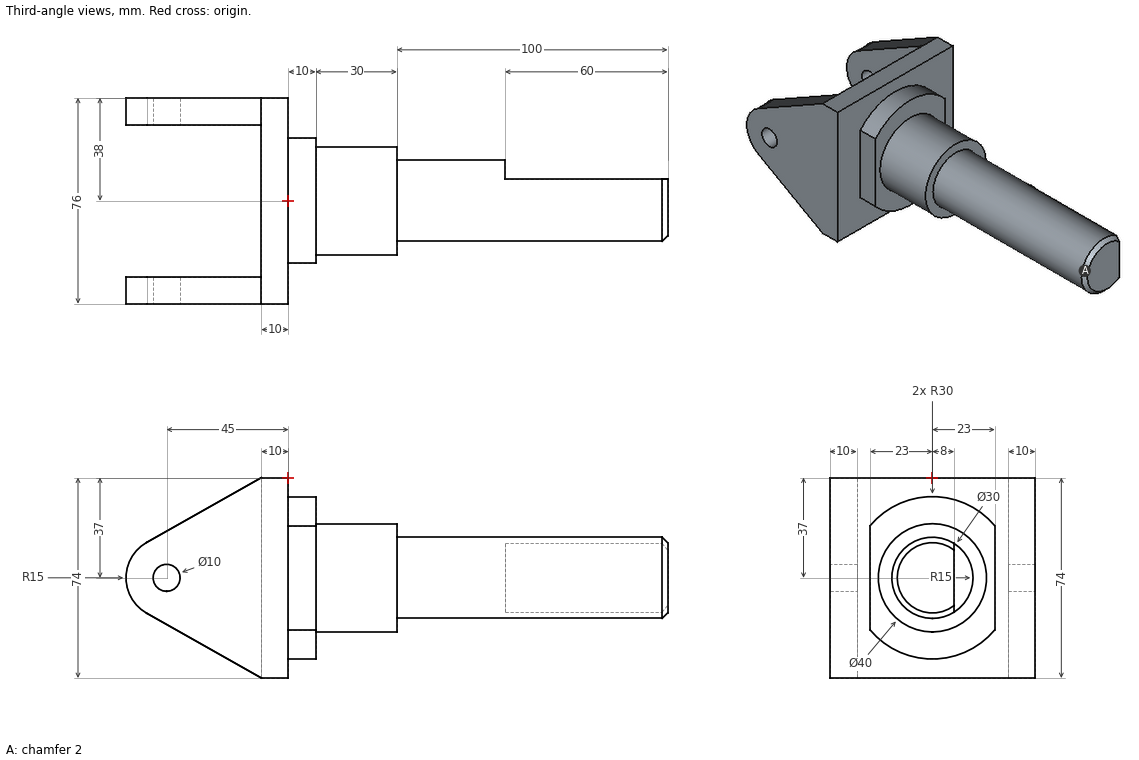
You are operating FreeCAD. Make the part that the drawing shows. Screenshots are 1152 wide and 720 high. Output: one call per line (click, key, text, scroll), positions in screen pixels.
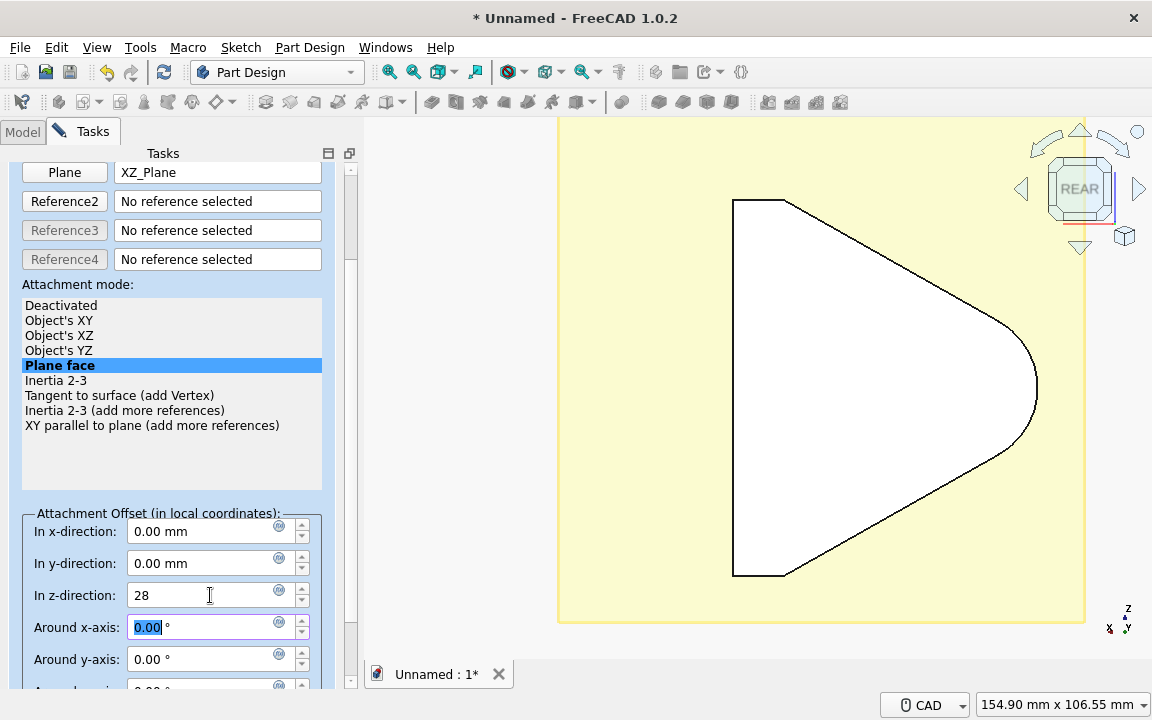
scroll(351, 426, up, 3)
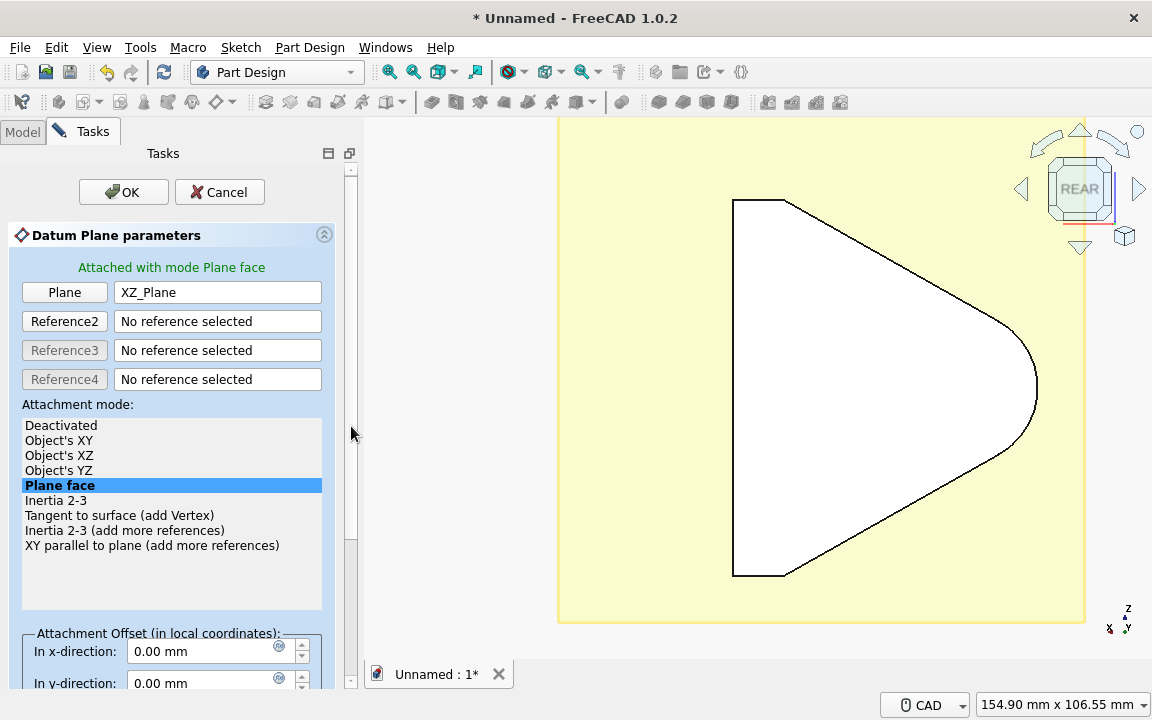
click(124, 192)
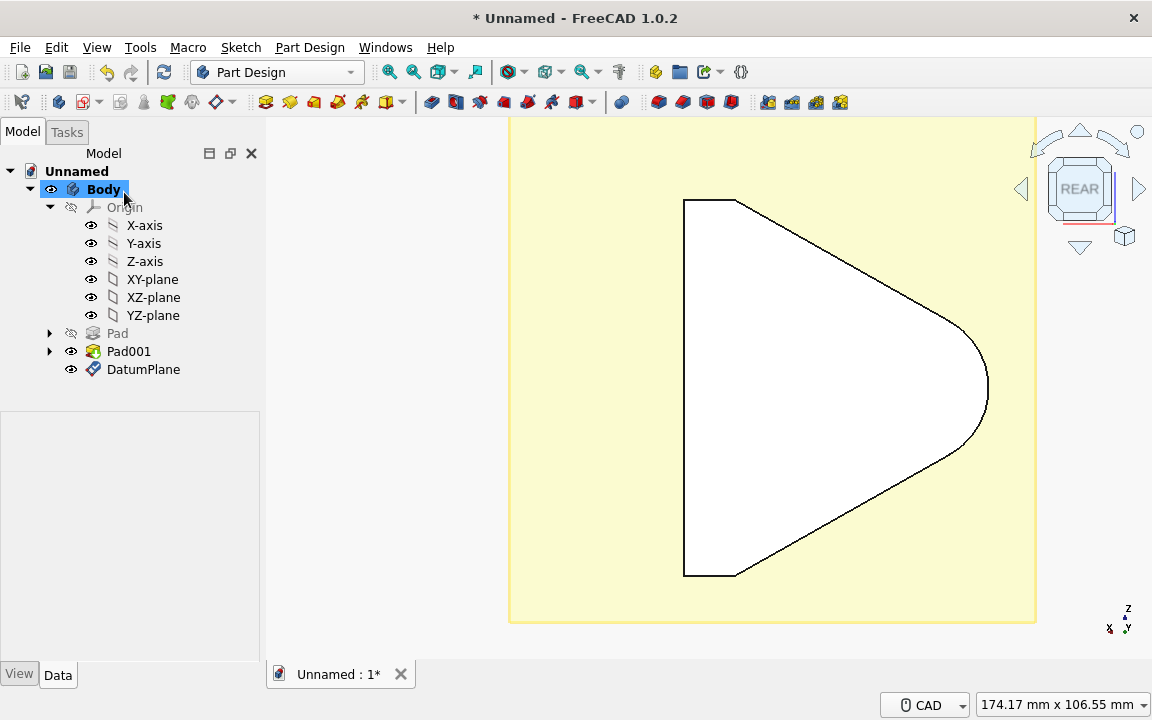
click(116, 369)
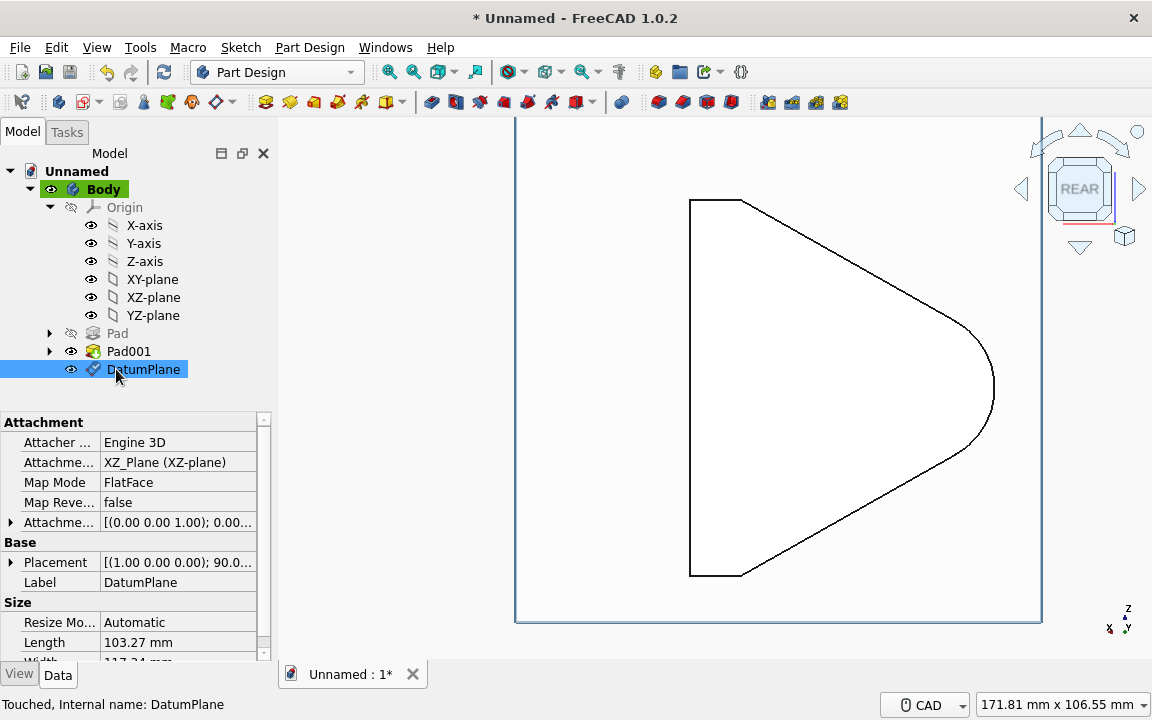
click(84, 102)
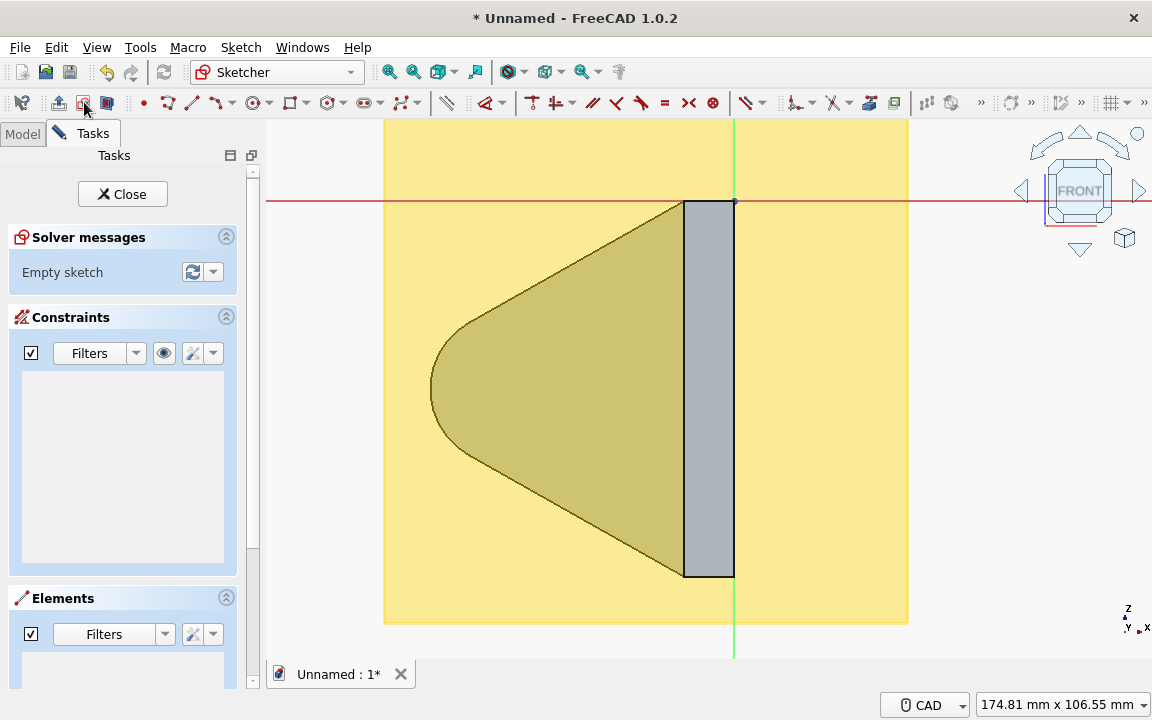
click(108, 104)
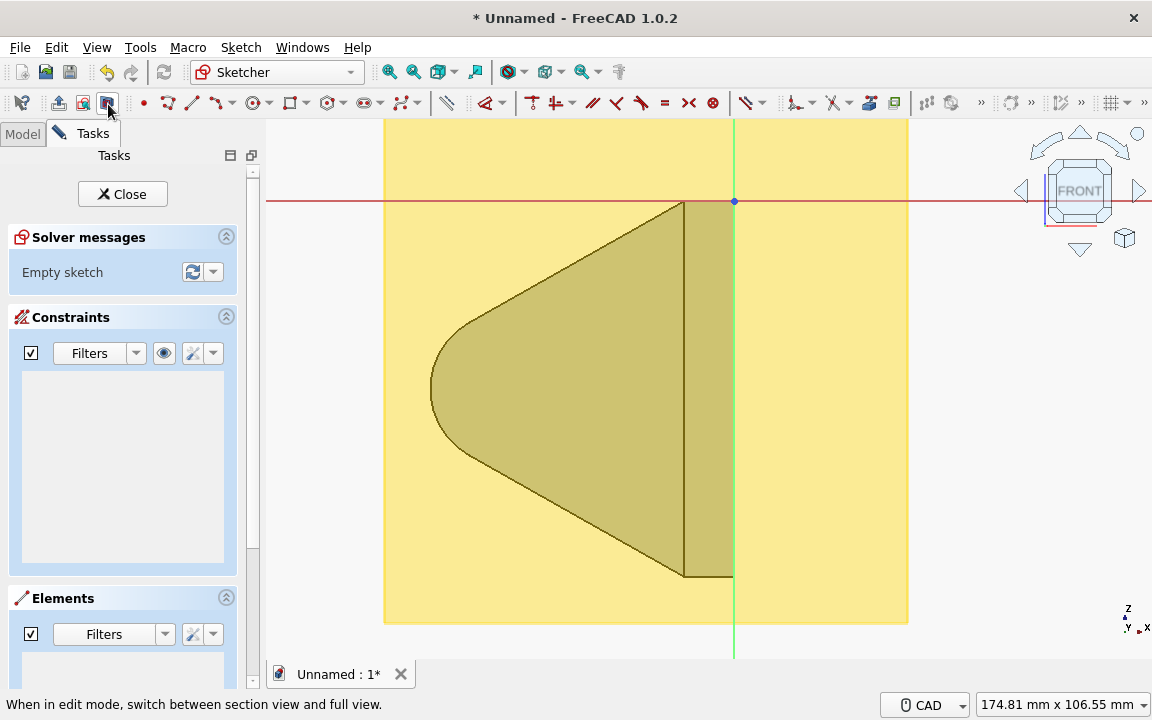
click(168, 104)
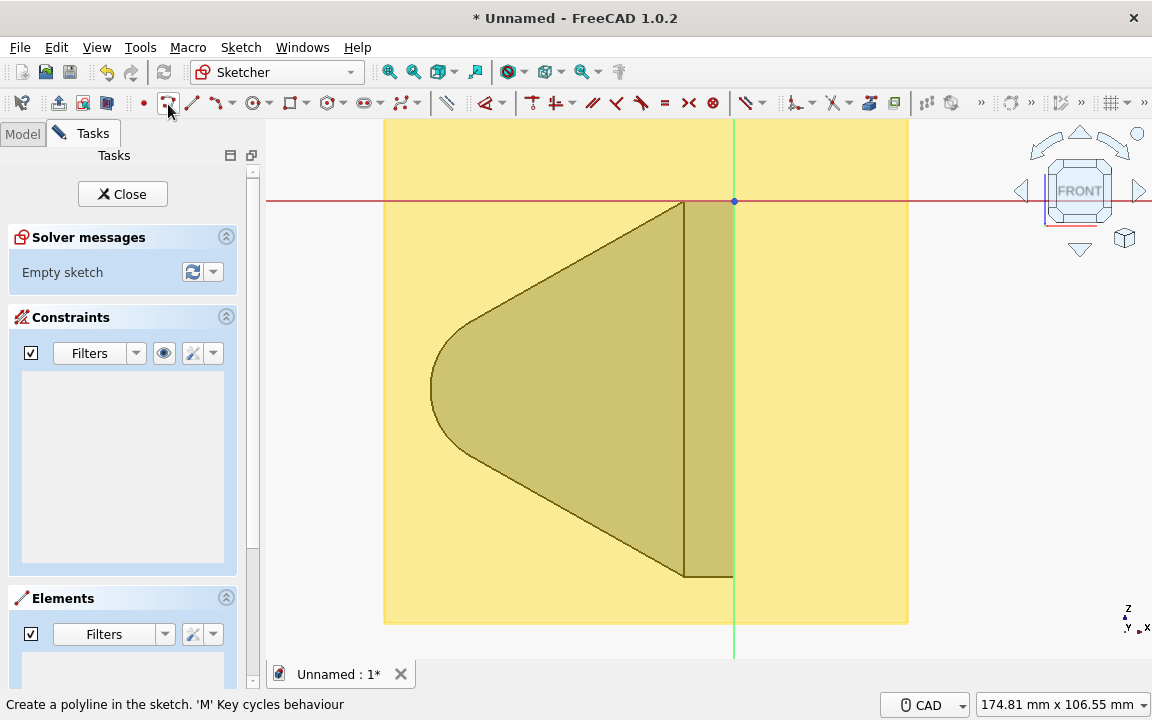
click(469, 455)
click(684, 577)
click(684, 201)
click(469, 323)
right_click(469, 323)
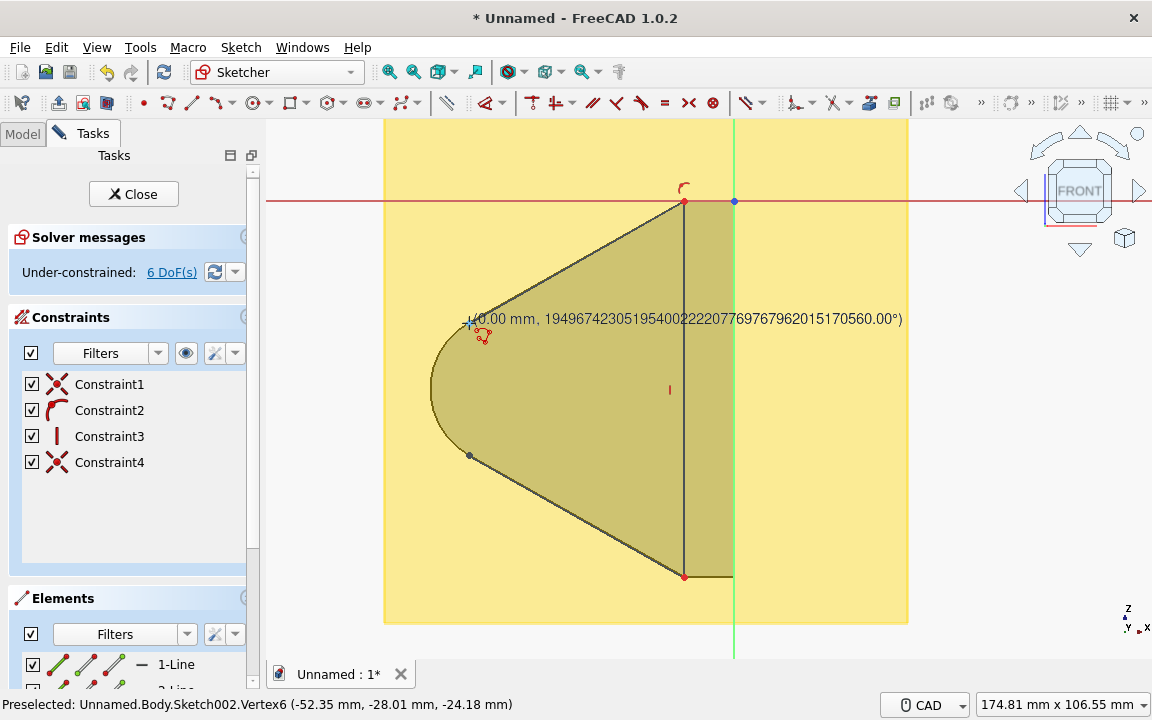
click(216, 104)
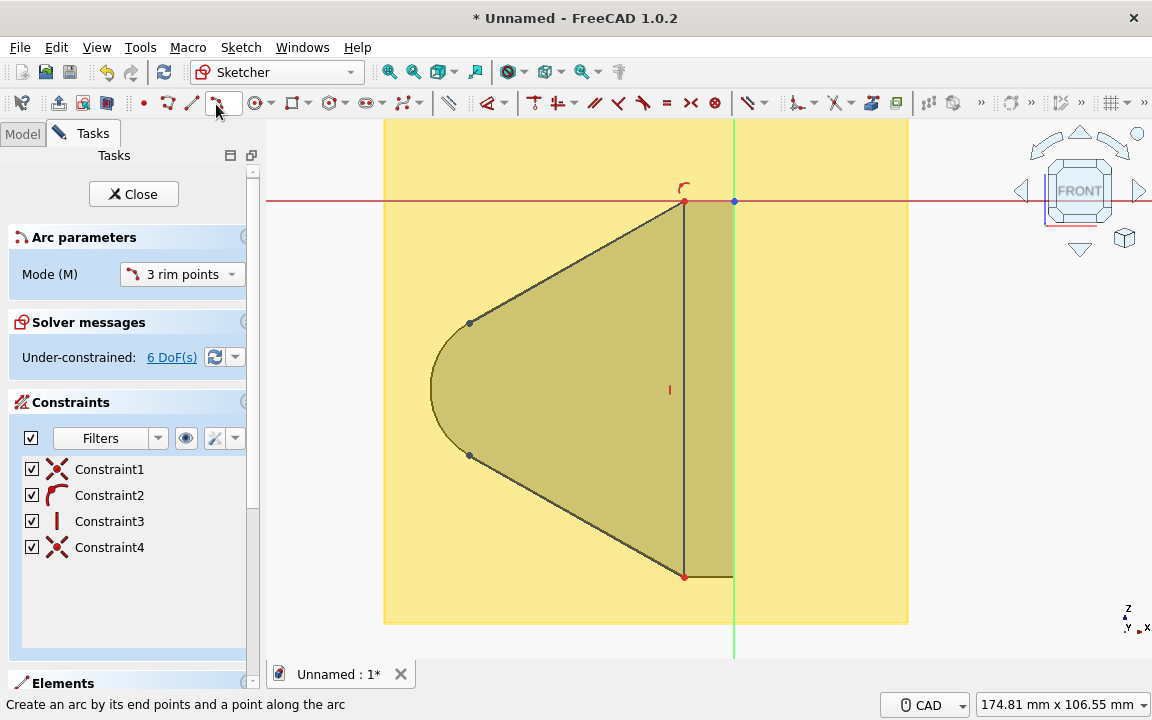
click(469, 324)
click(469, 456)
click(430, 389)
key(Escape)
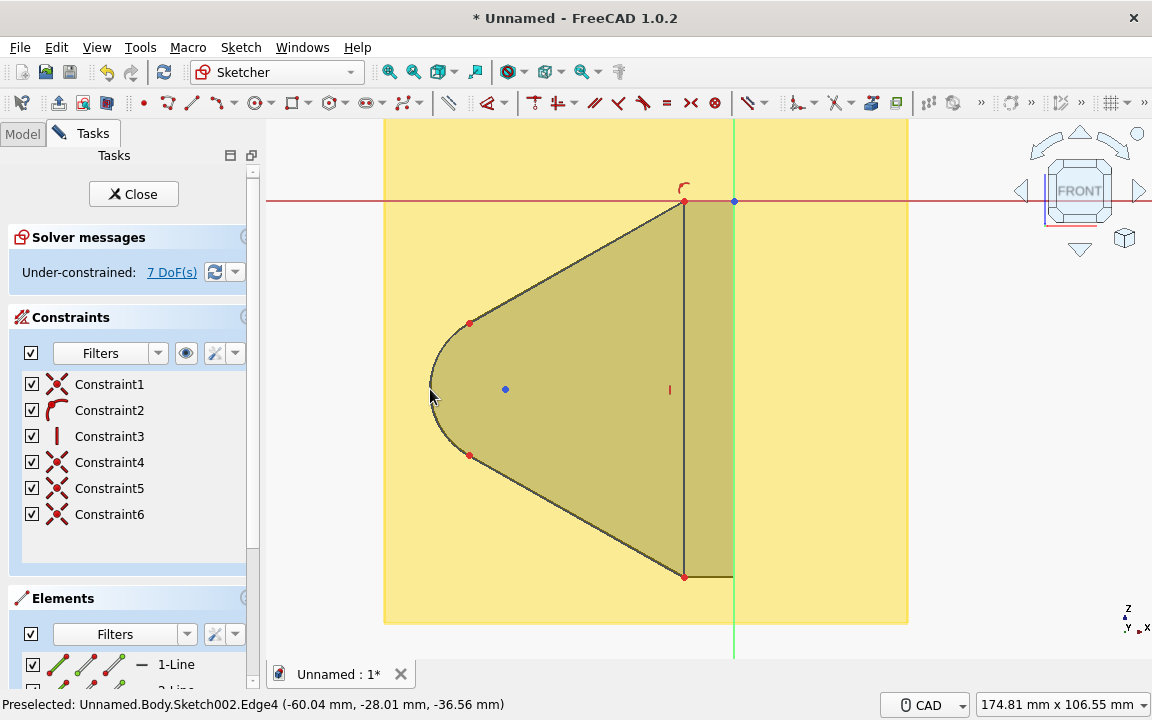
click(534, 493)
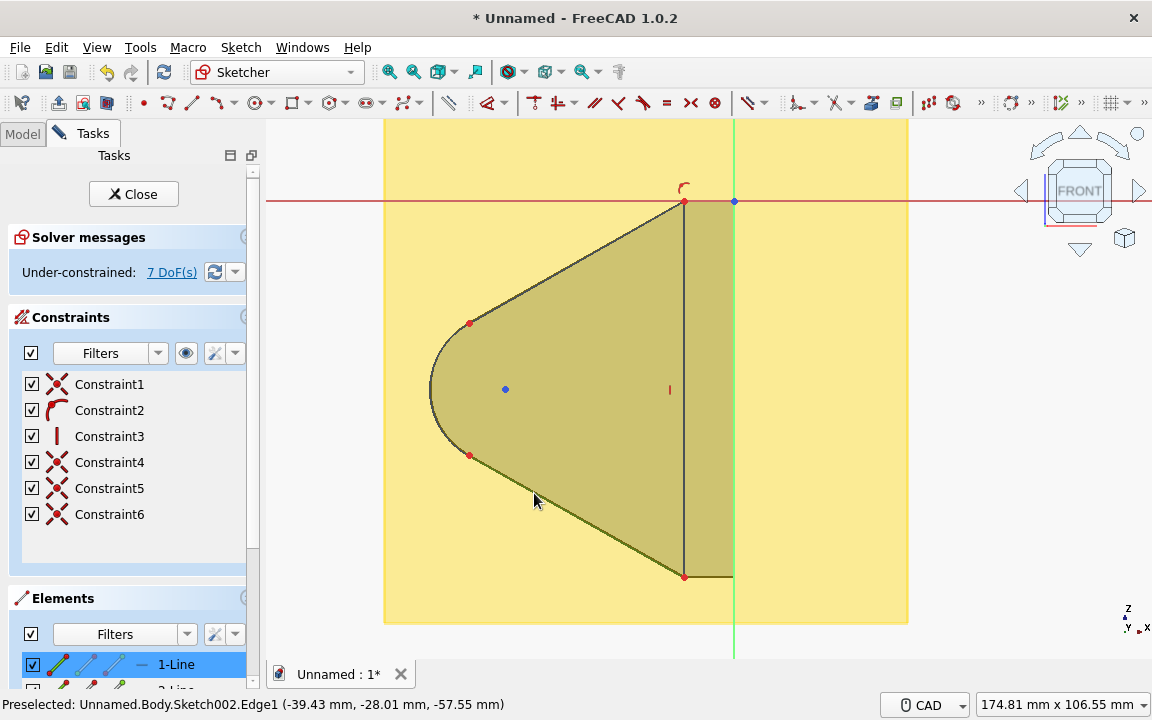
click(437, 359)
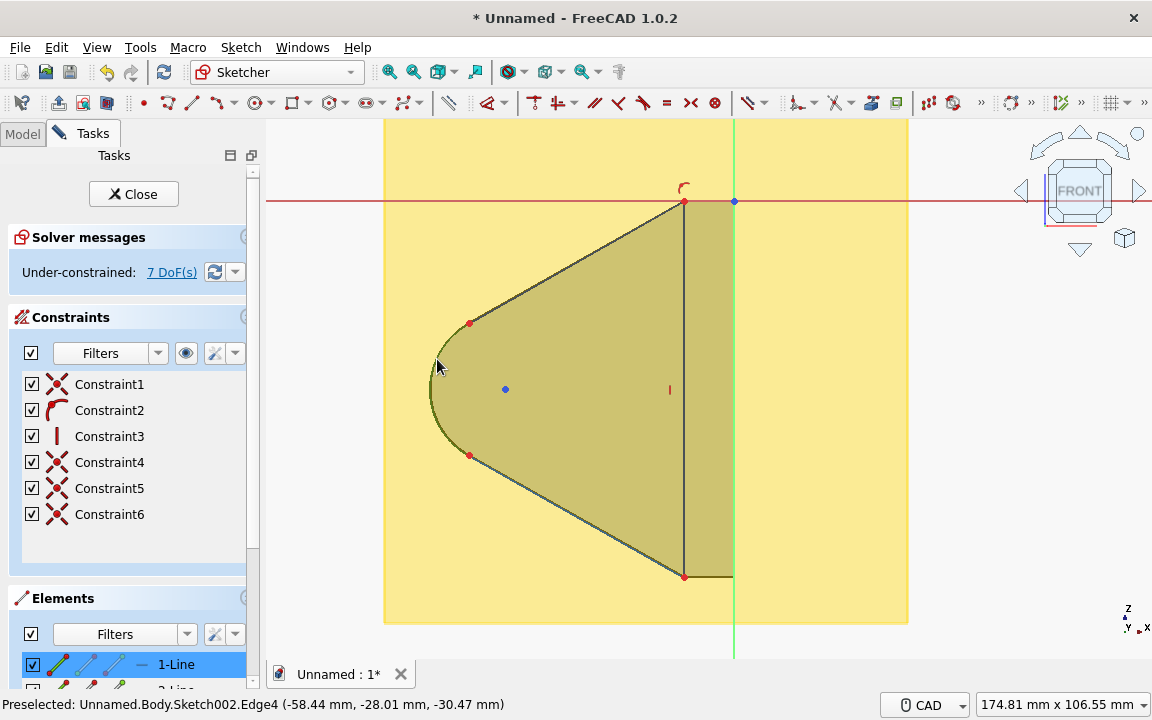
click(644, 104)